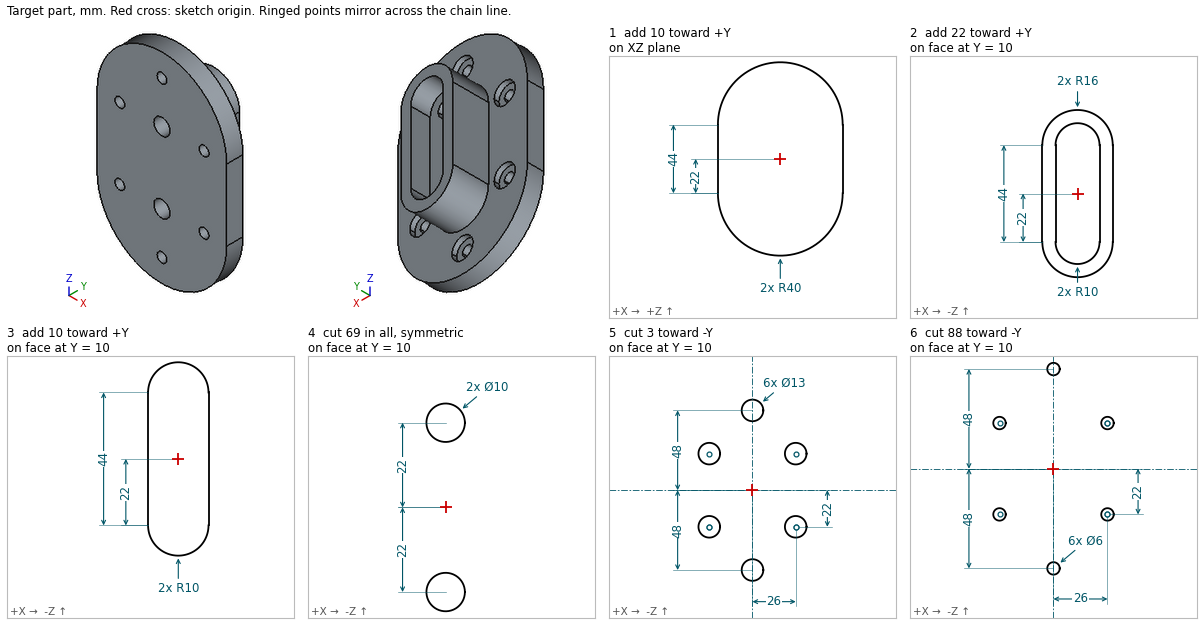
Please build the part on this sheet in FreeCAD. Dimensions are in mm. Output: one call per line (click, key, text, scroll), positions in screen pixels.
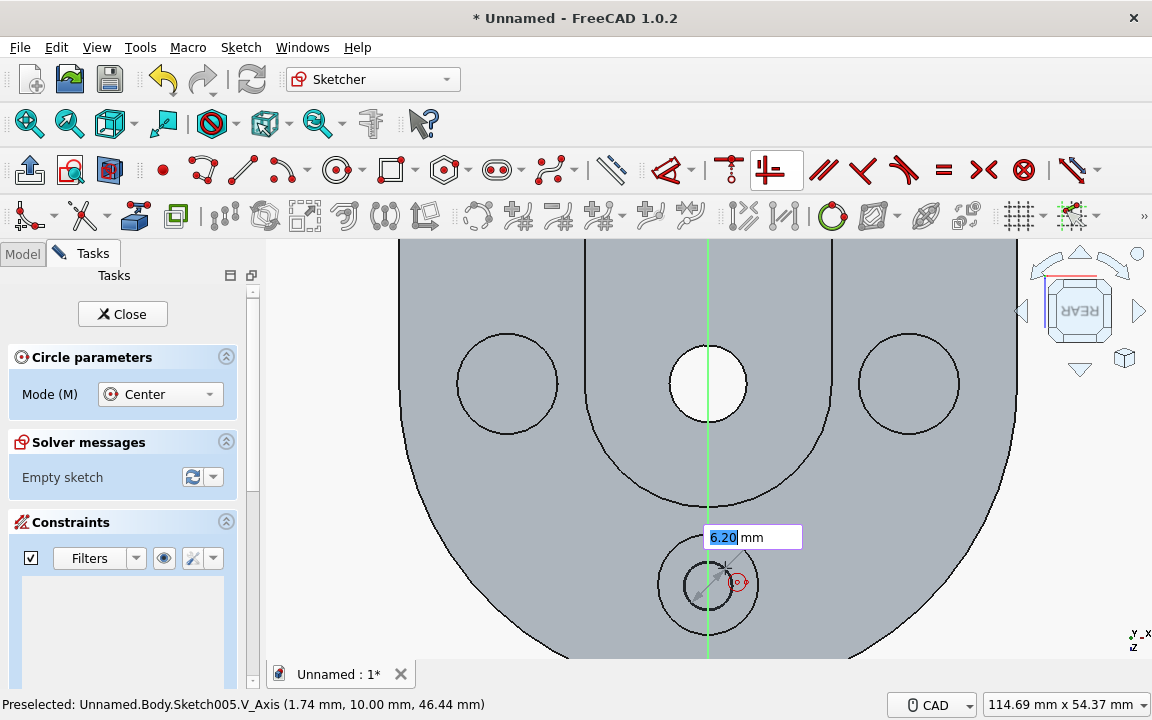
text(6)
key(Return)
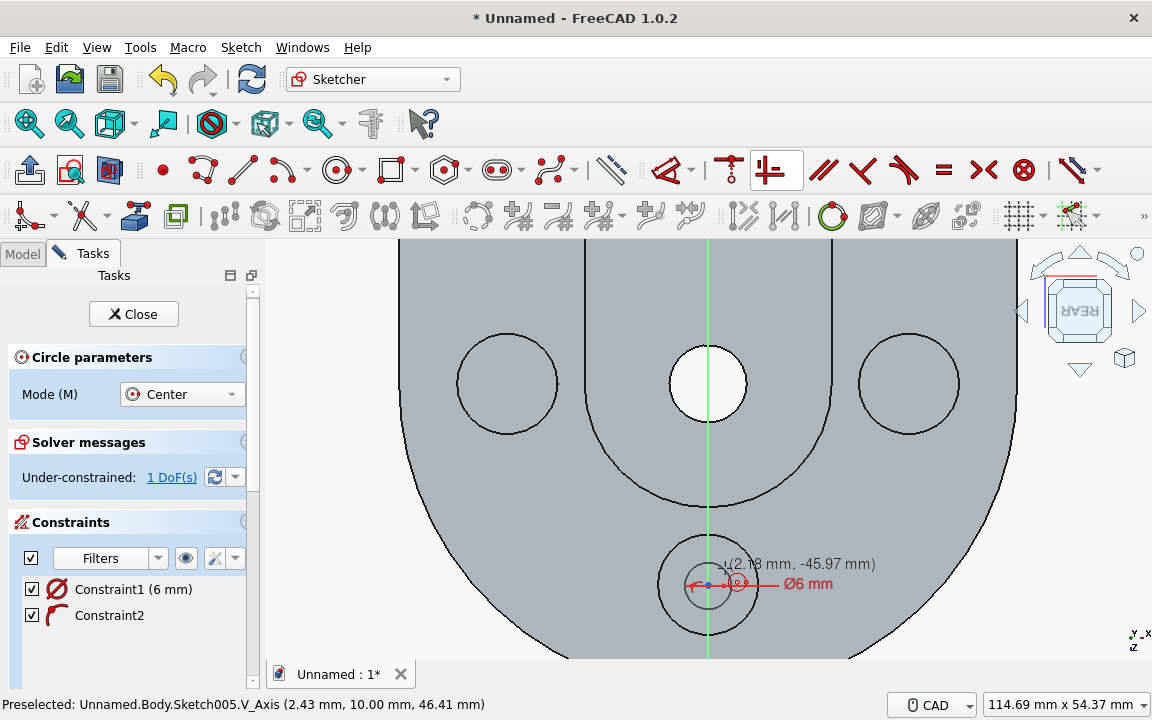
click(909, 384)
move(925, 367)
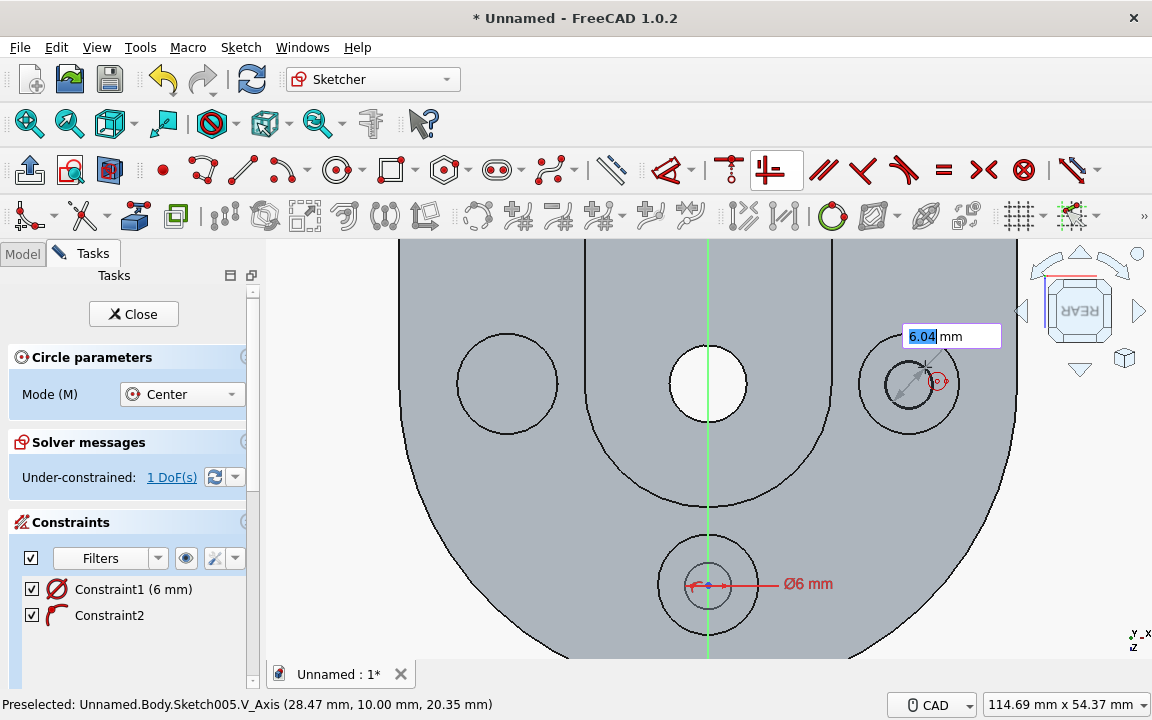
text(6)
key(Return)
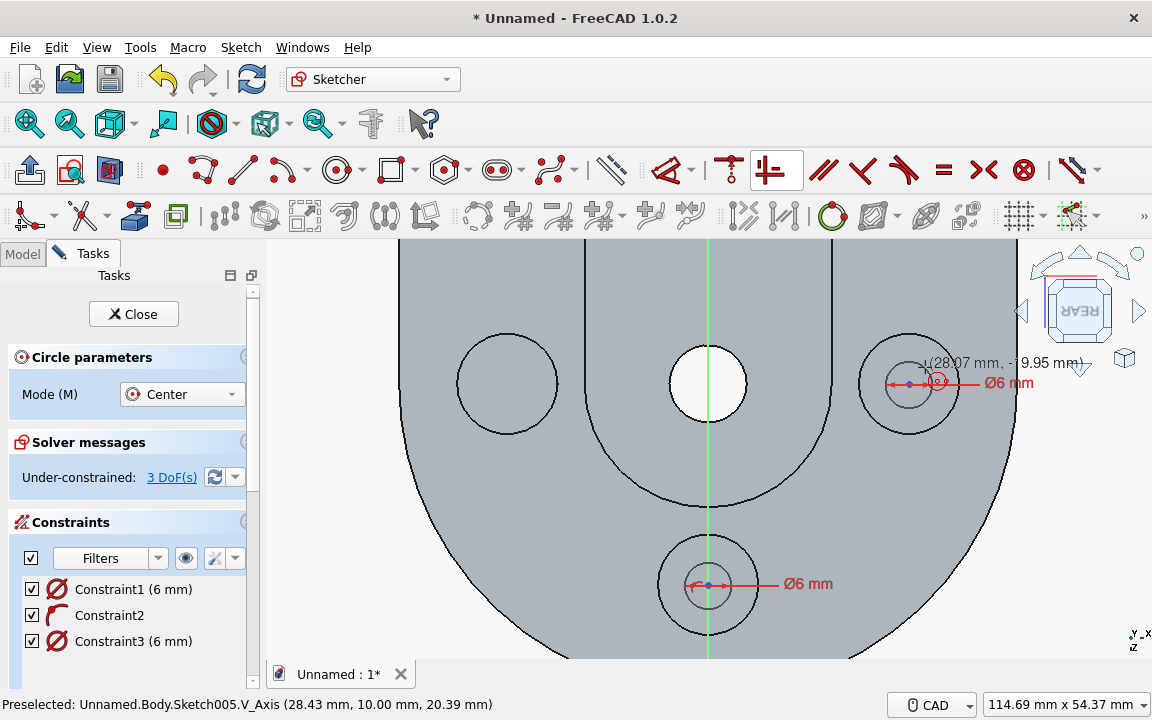
scroll(611, 550, down, 6)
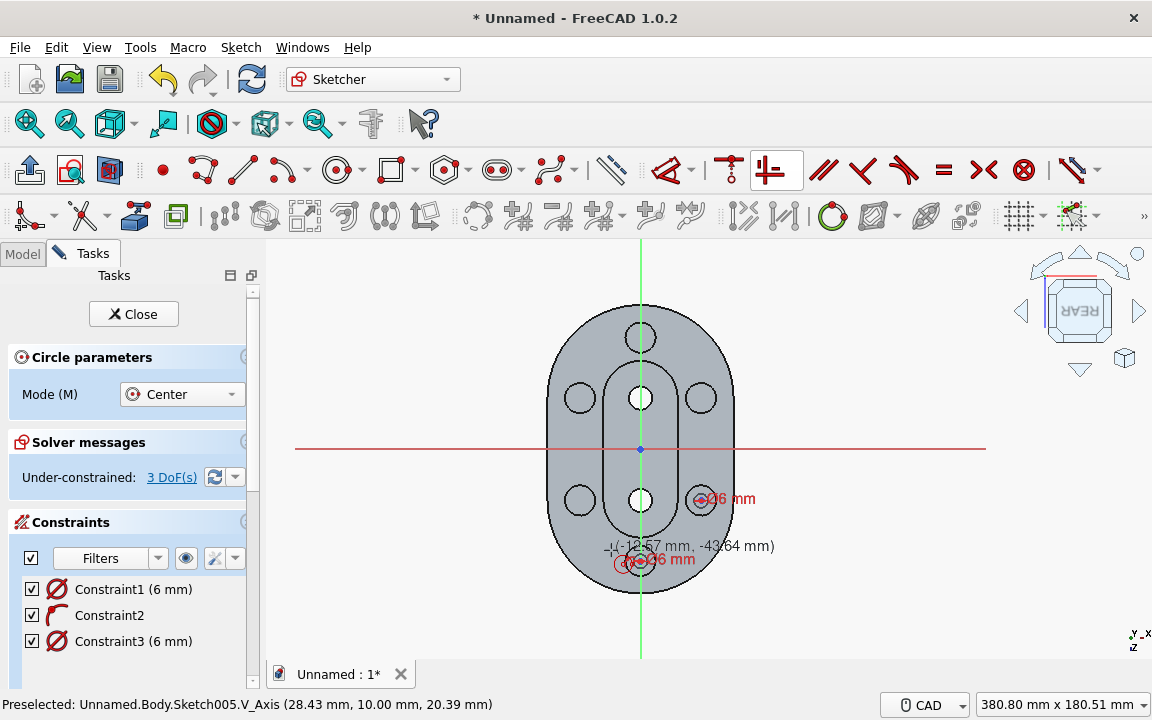
scroll(701, 398, up, 6)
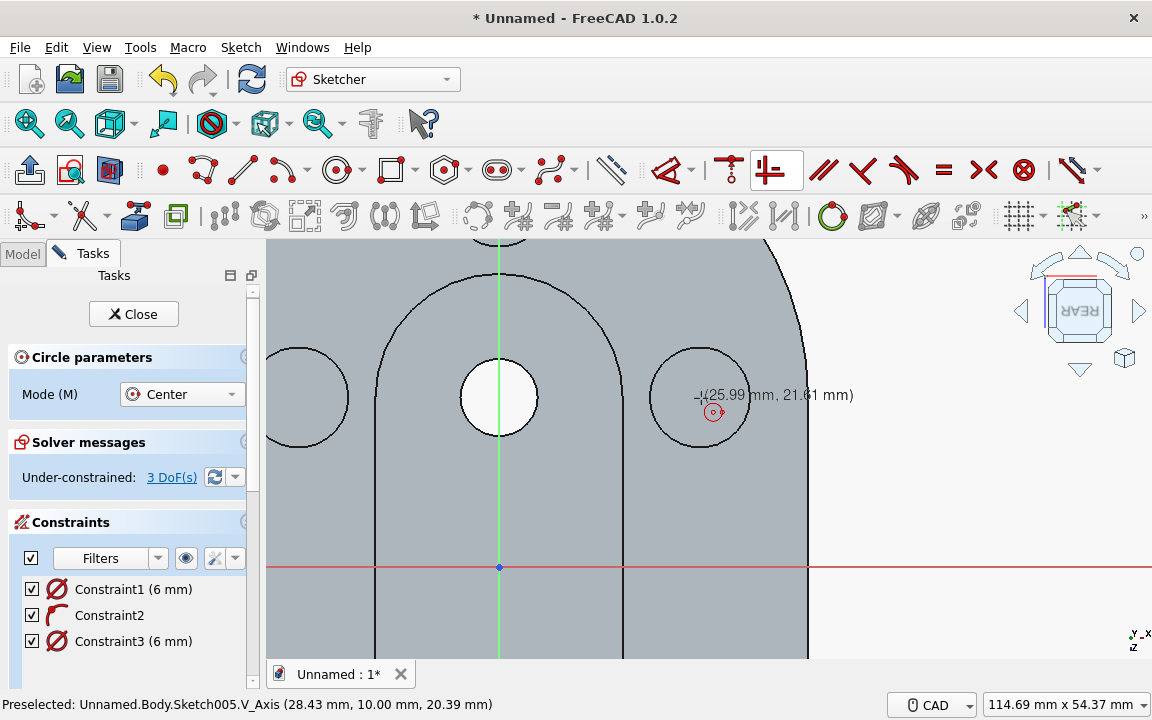
click(700, 397)
move(716, 381)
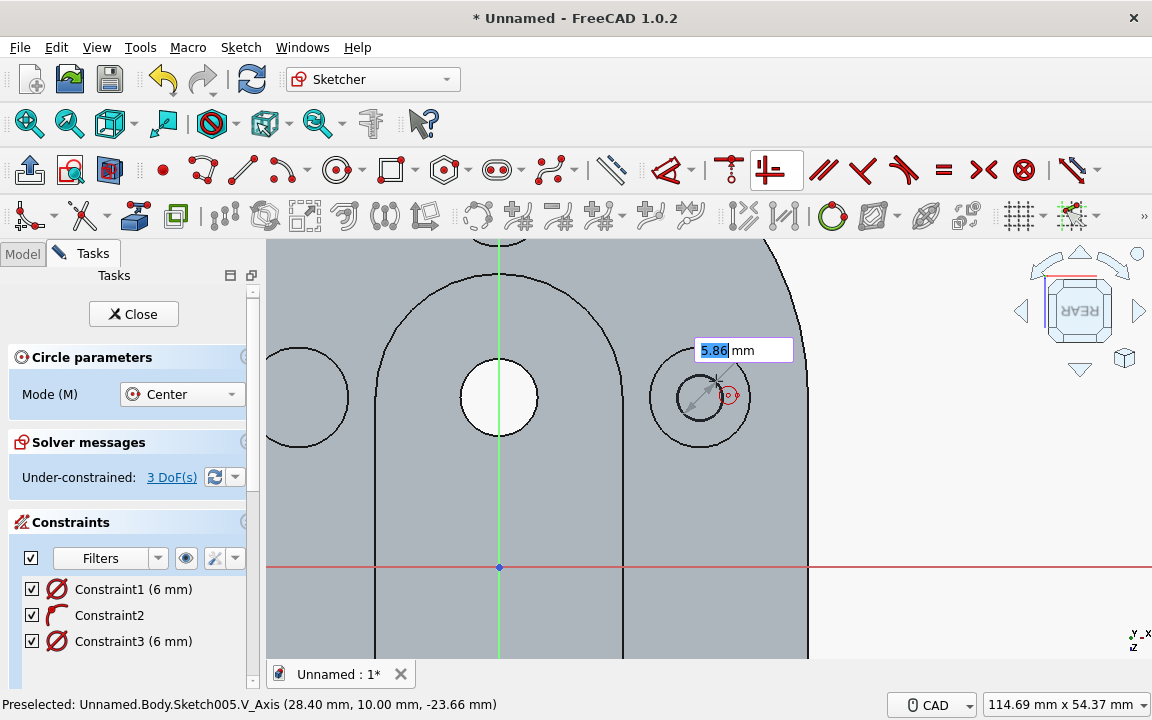
text(6)
key(Return)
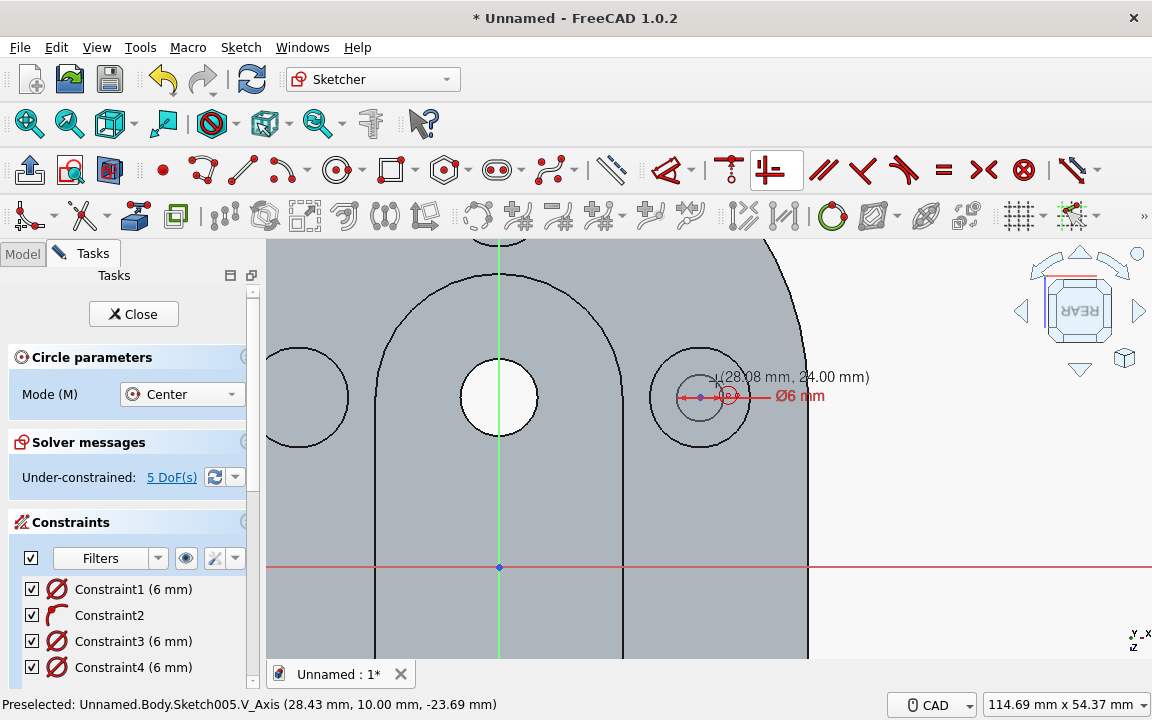
scroll(701, 398, down, 6)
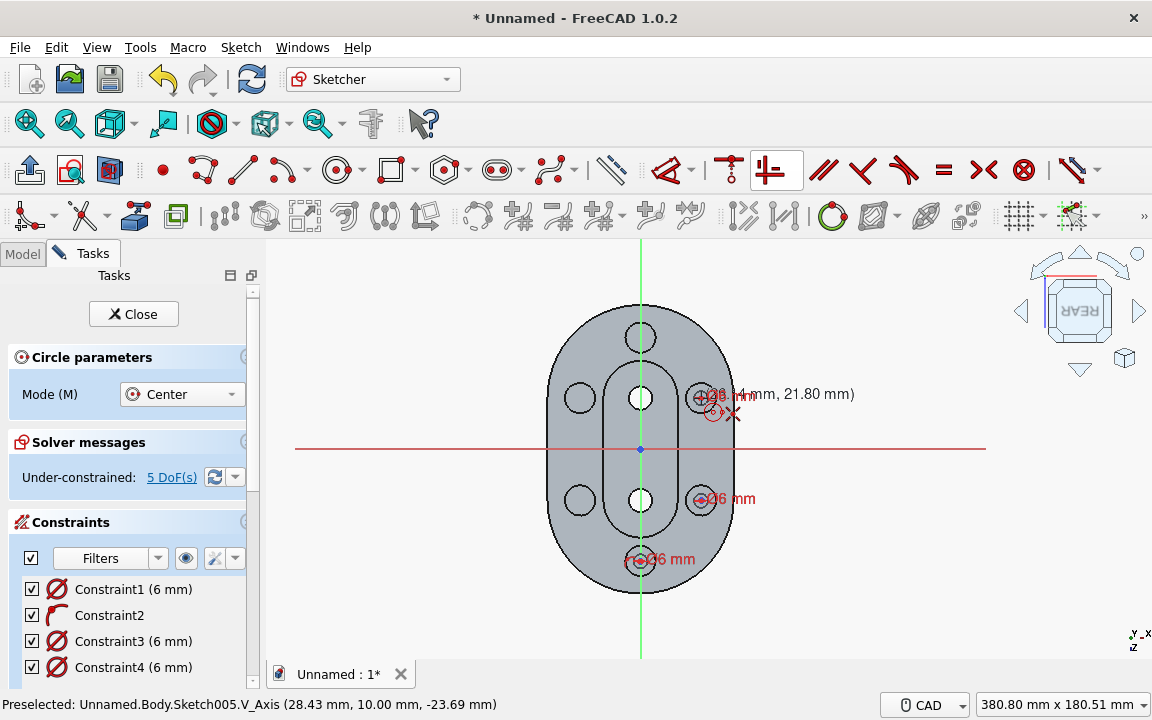
scroll(641, 338, up, 6)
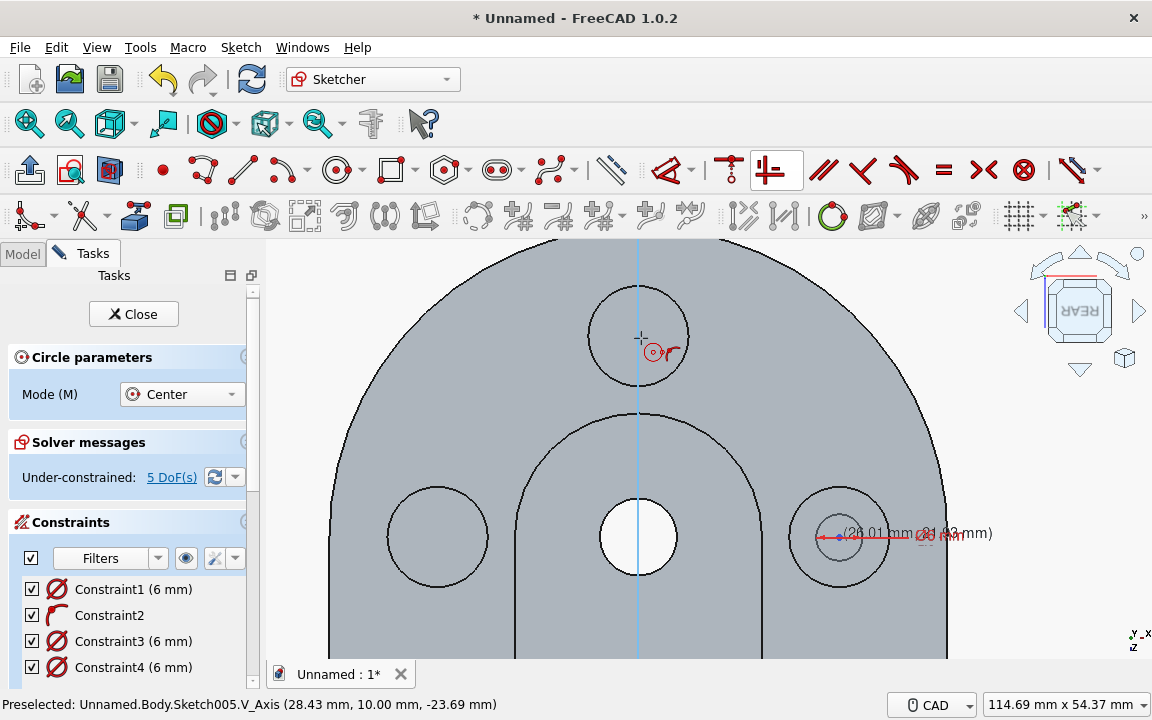
click(638, 336)
move(655, 320)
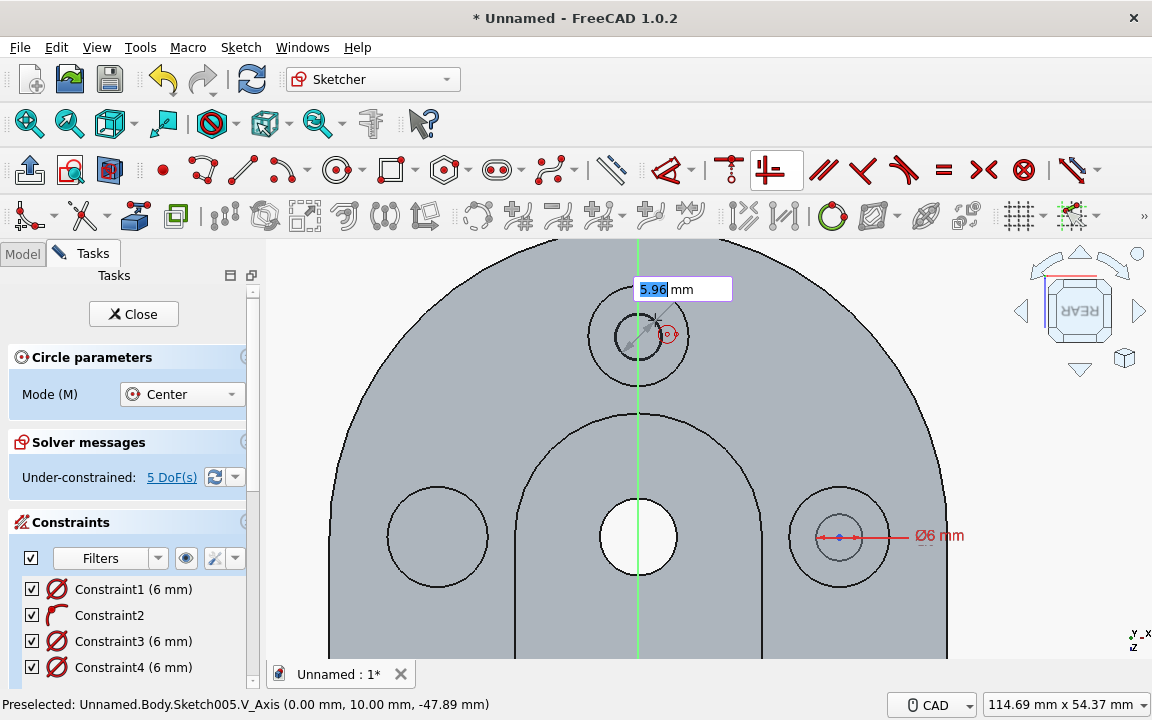
text(6)
key(Return)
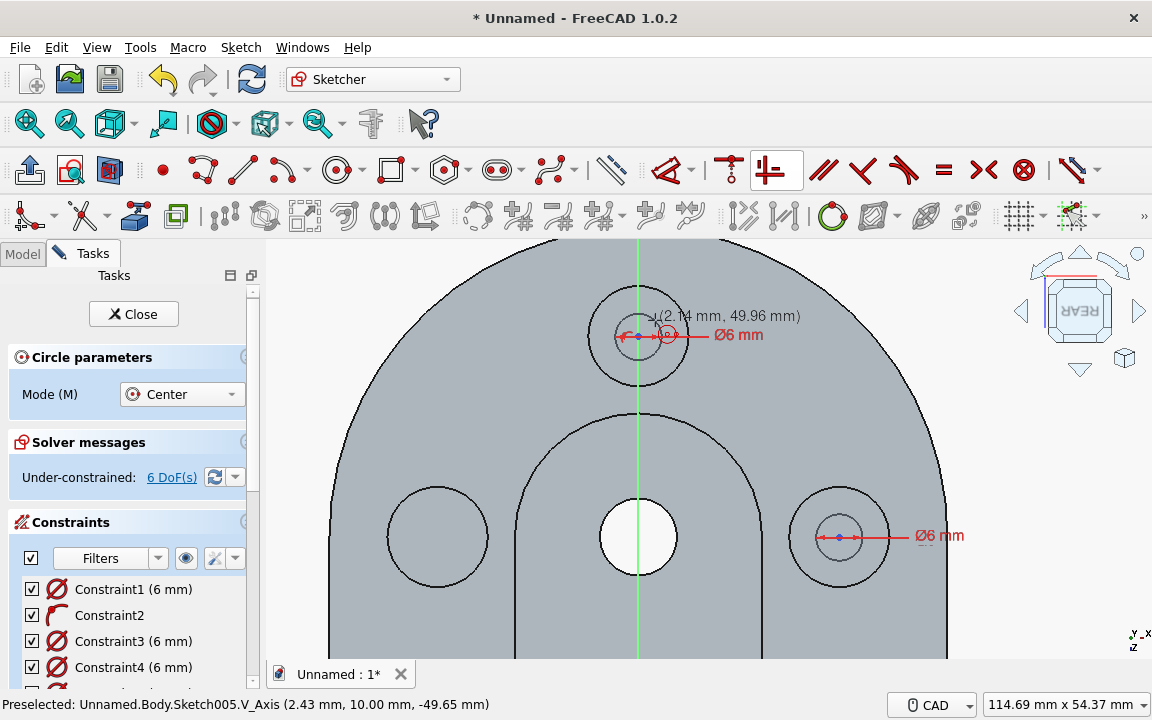
click(438, 537)
move(454, 521)